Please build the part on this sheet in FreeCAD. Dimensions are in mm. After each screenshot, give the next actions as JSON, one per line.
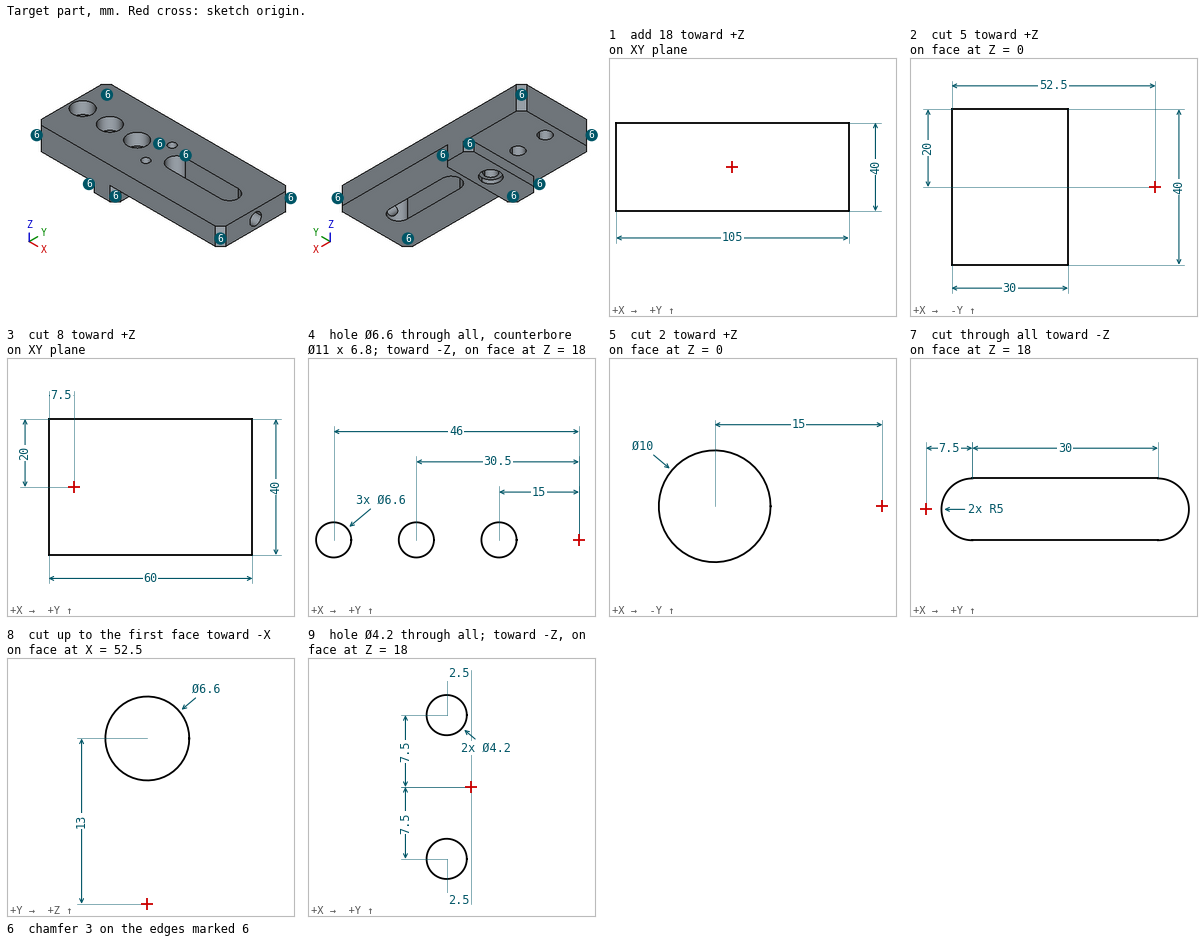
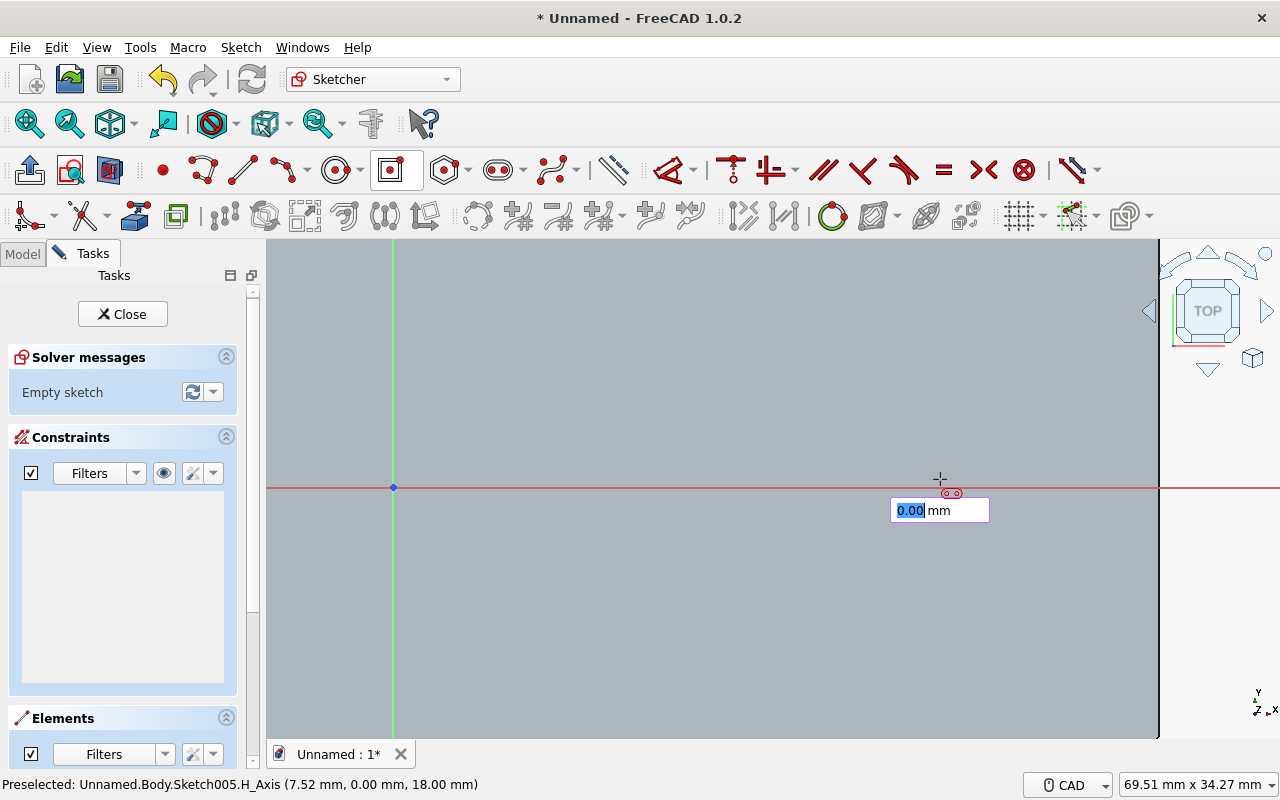
{"action": "left_click", "coordinate": [722, 415]}
{"action": "key", "text": "Escape"}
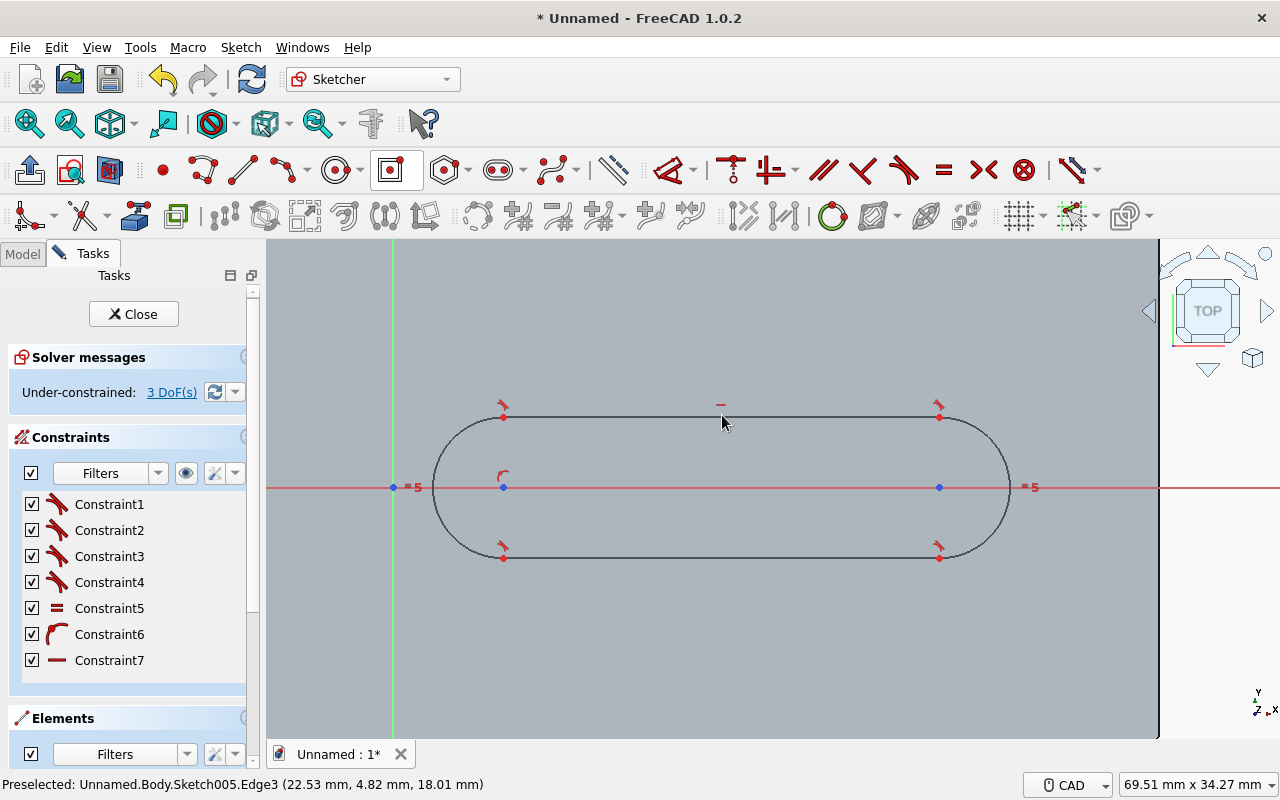
{"action": "key", "text": "d"}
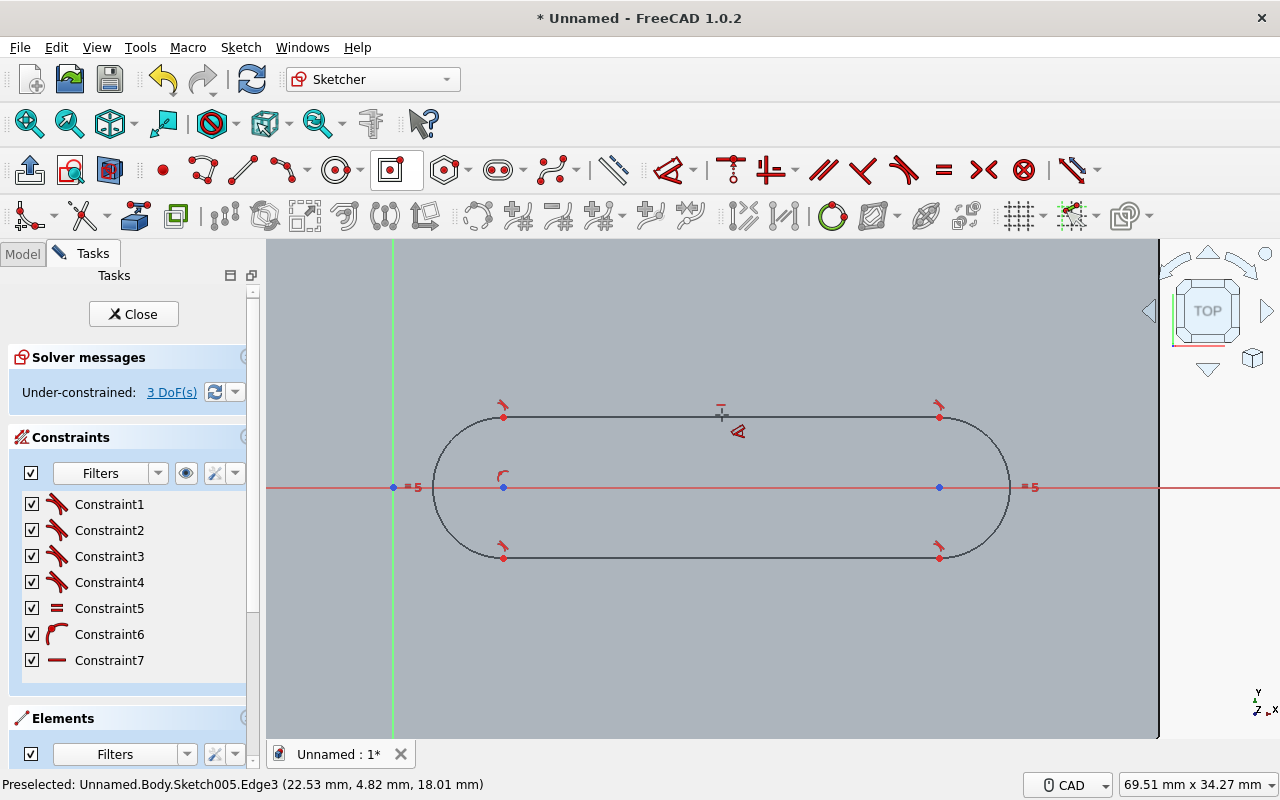
{"action": "left_click", "coordinate": [446, 446]}
{"action": "left_click", "coordinate": [420, 427]}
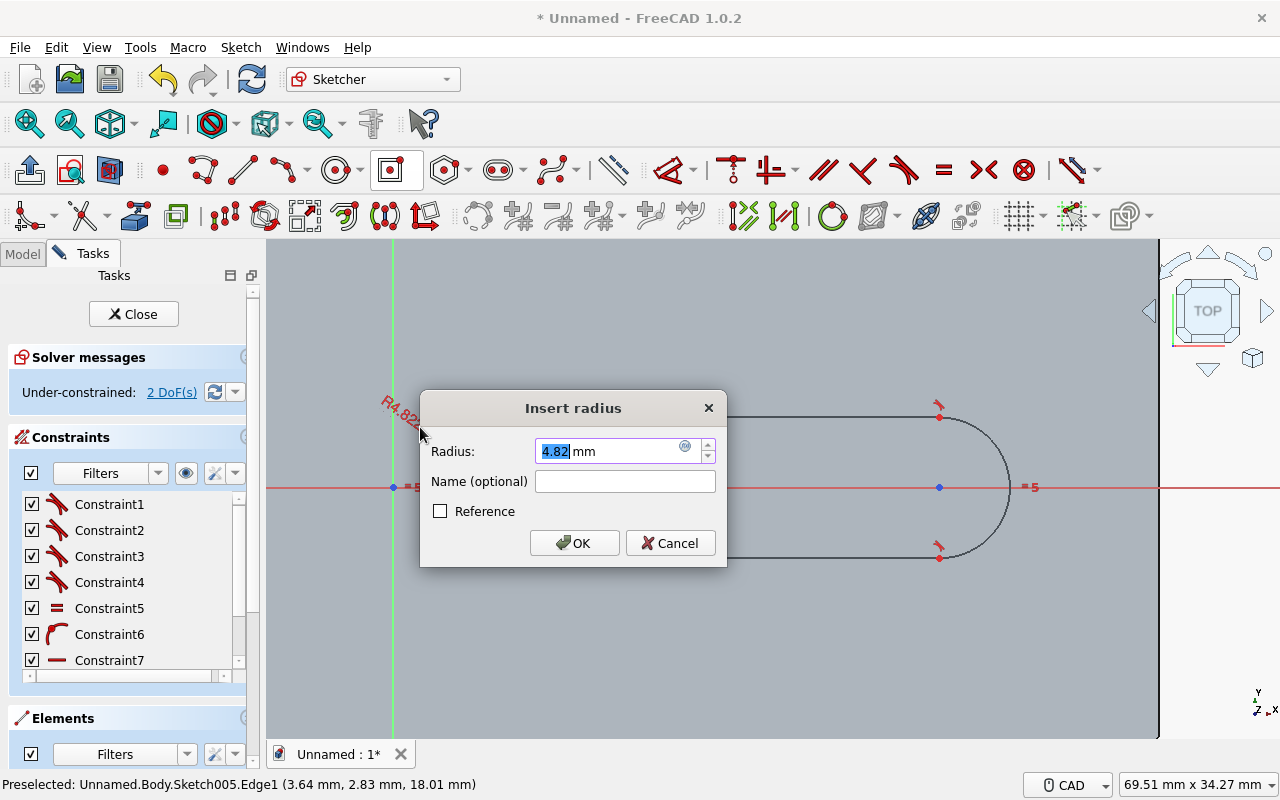
{"action": "type", "text": "5"}
{"action": "key", "text": "Return"}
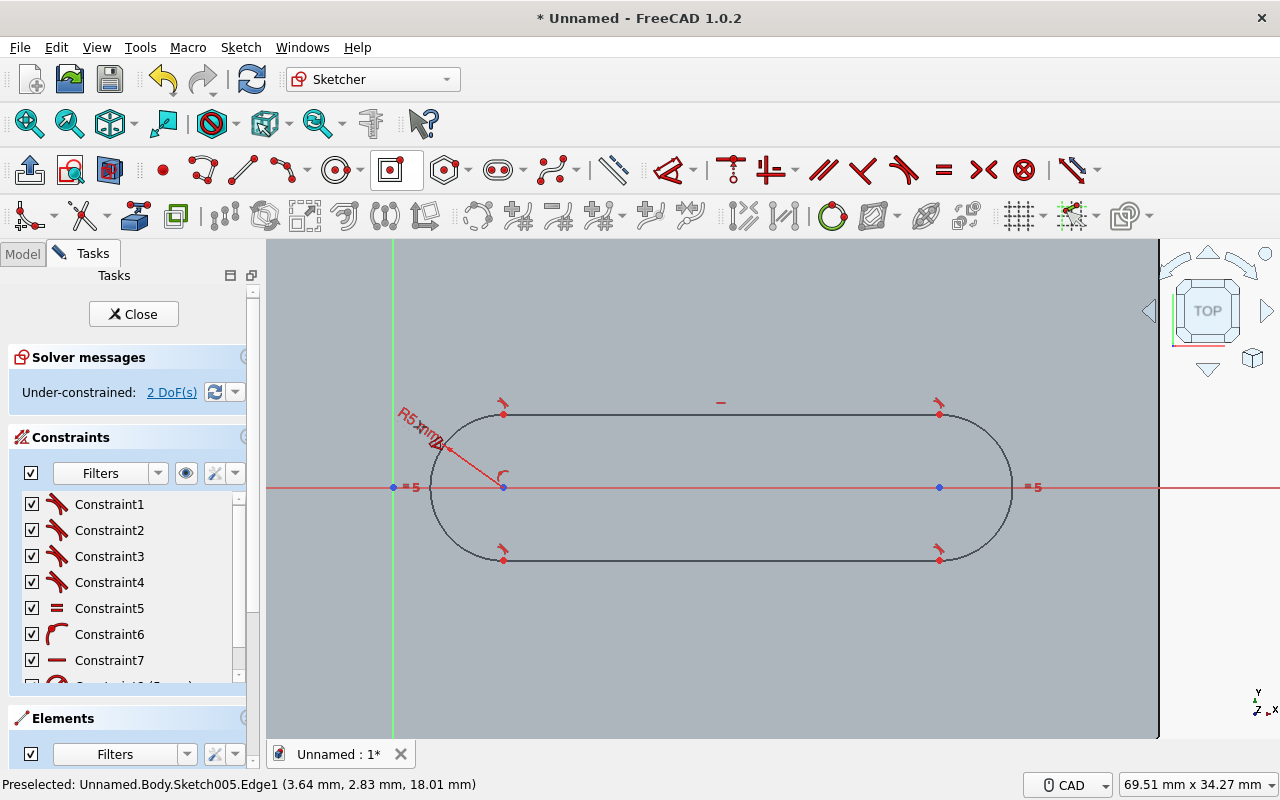
{"action": "left_click", "coordinate": [634, 415]}
{"action": "left_click", "coordinate": [721, 381]}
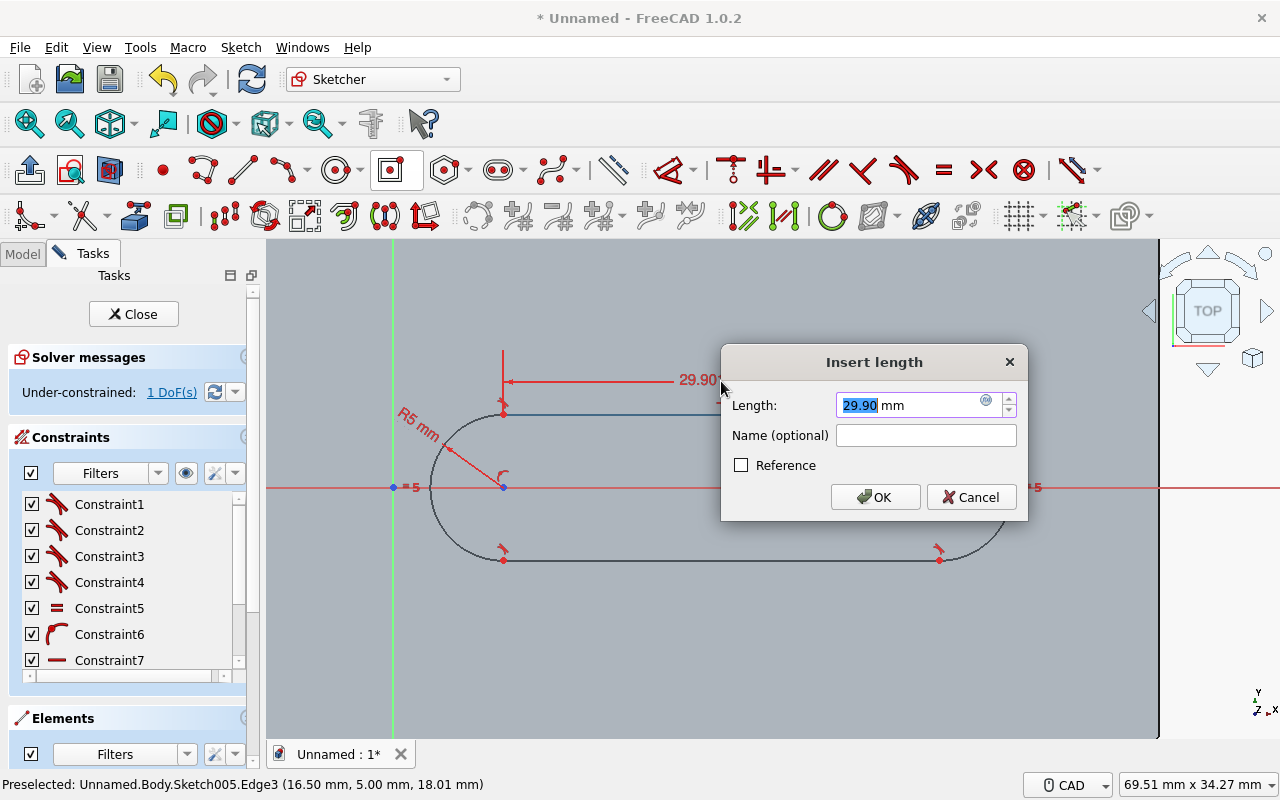
{"action": "type", "text": "30"}
{"action": "key", "text": "Return"}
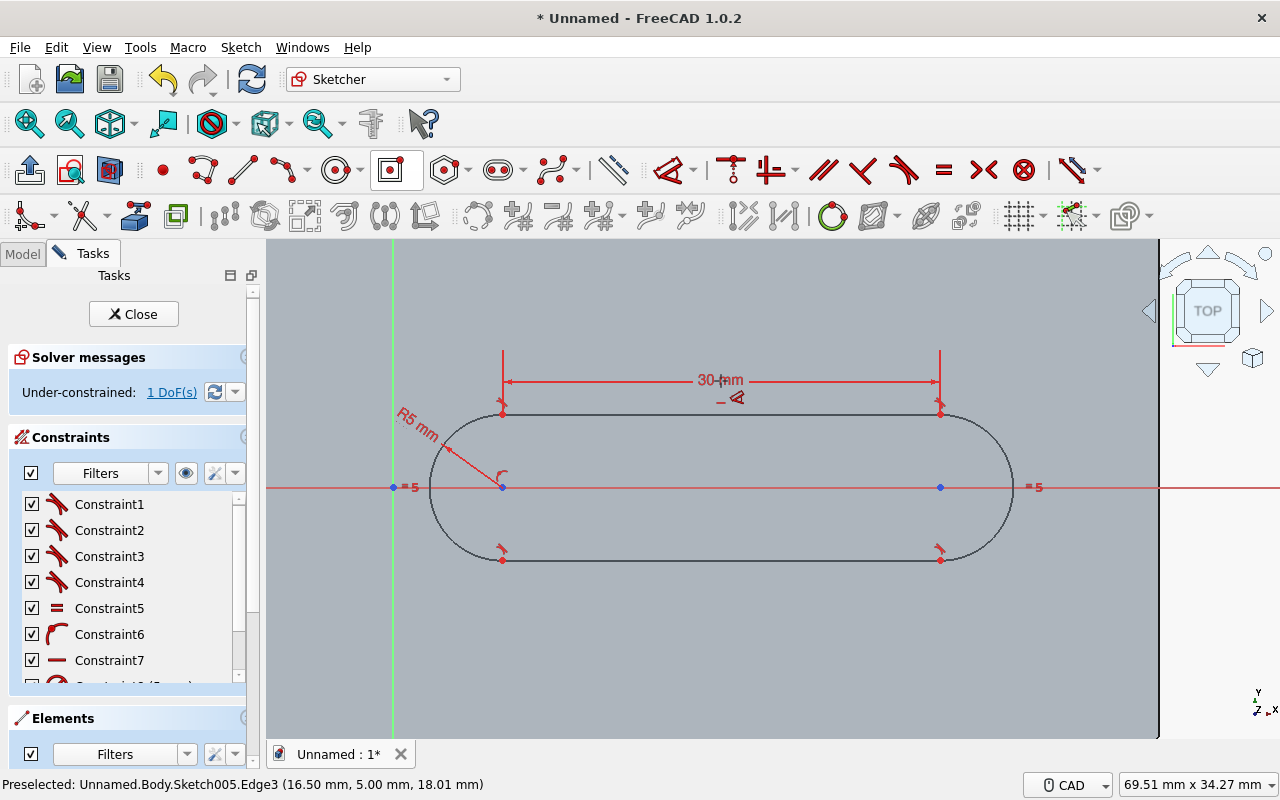
{"action": "left_click", "coordinate": [503, 415]}
{"action": "left_click", "coordinate": [448, 381]}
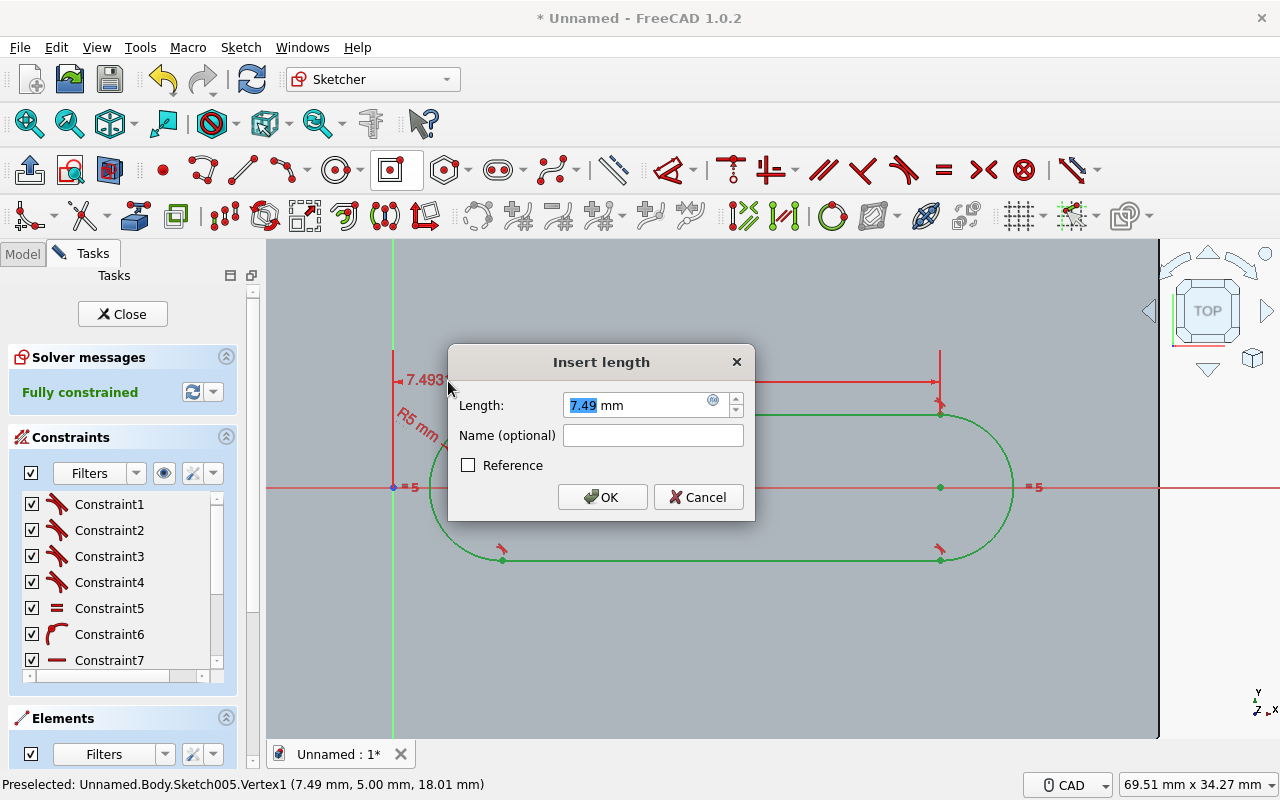
{"action": "type", "text": "7.5"}
{"action": "key", "text": "Return"}
{"action": "key", "text": "Escape"}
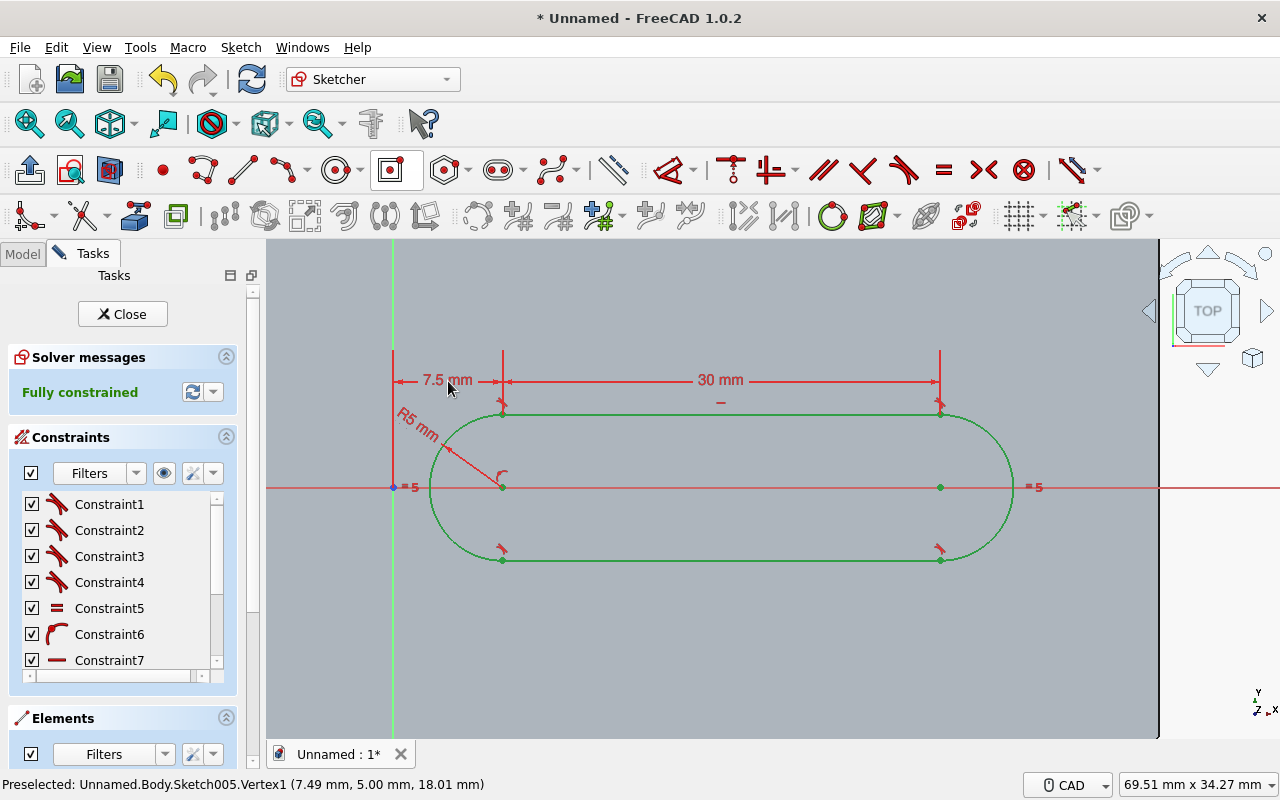
{"action": "left_click", "coordinate": [123, 314]}